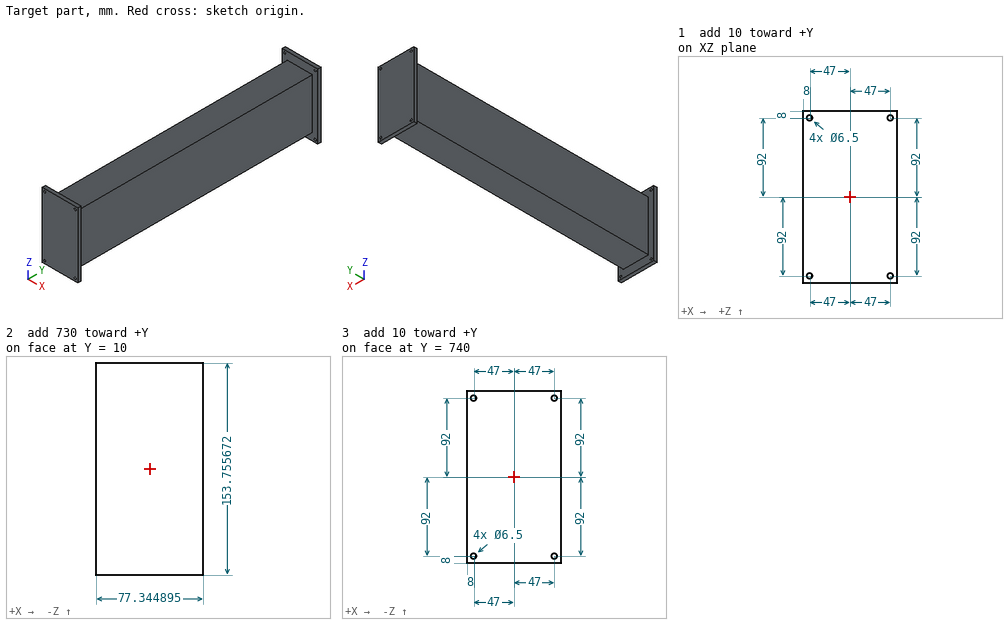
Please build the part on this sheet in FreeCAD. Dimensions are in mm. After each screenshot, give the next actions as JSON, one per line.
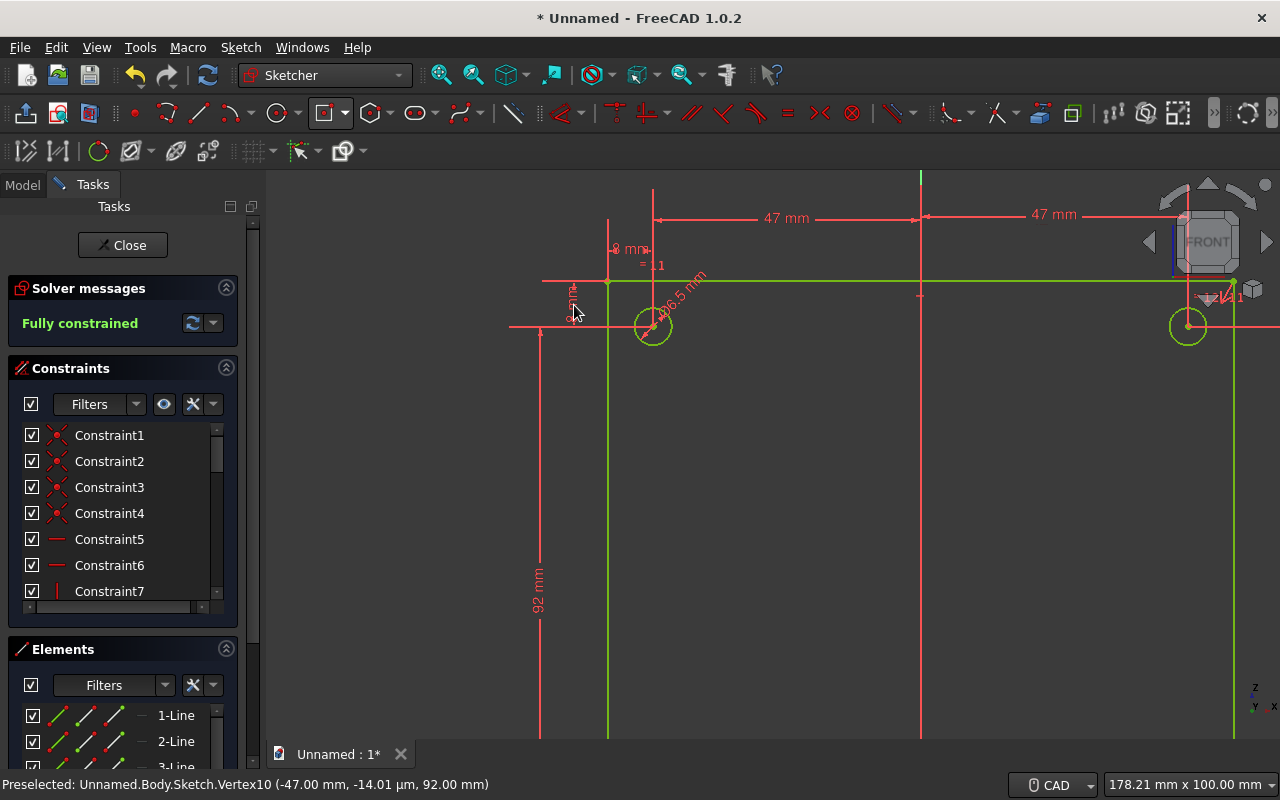
{"action": "left_click", "coordinate": [123, 245]}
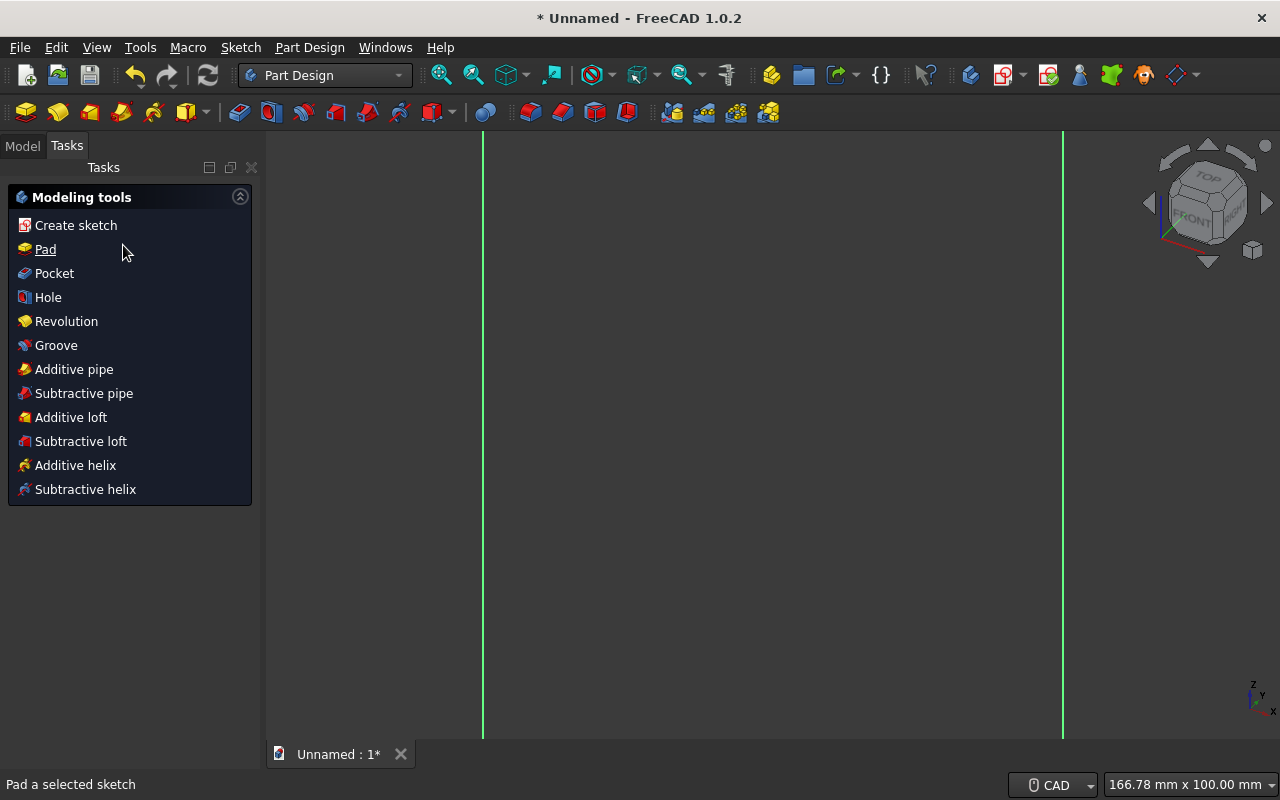
{"action": "left_click", "coordinate": [26, 112]}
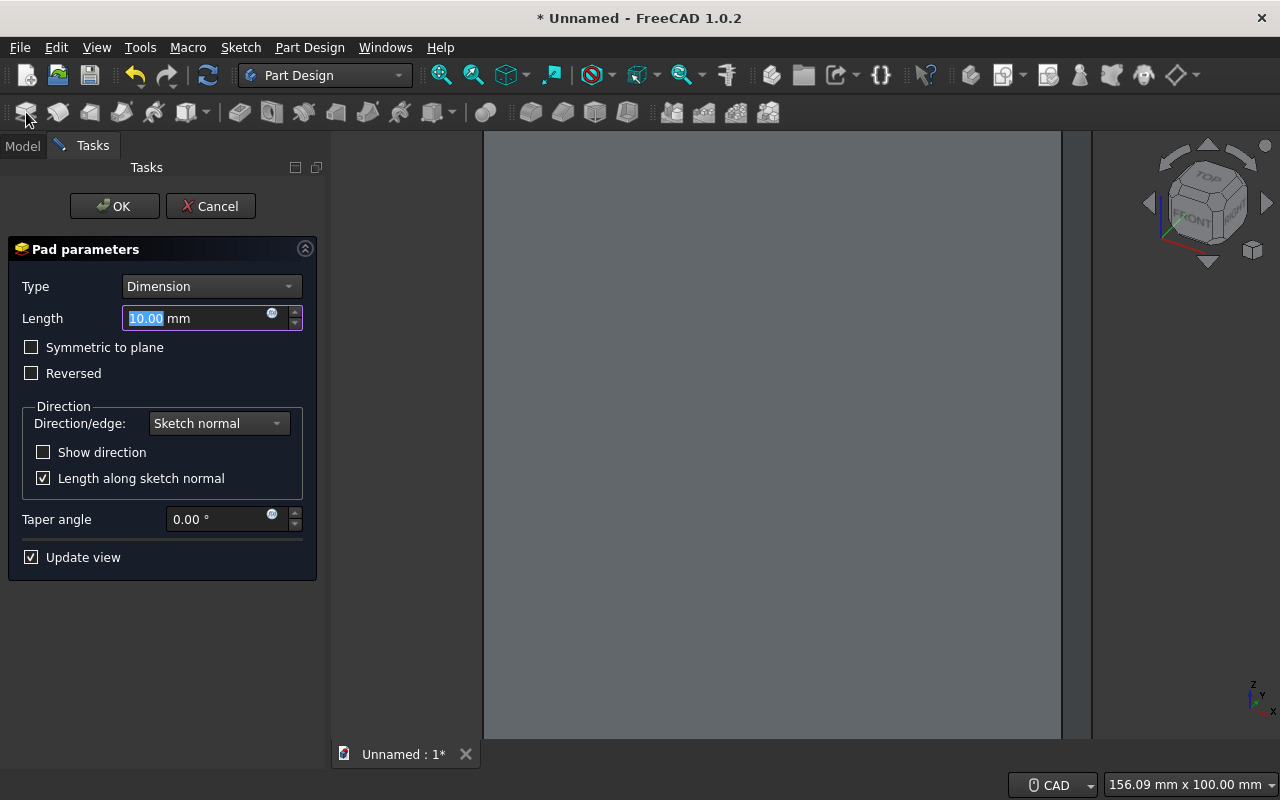
{"action": "type", "text": "10"}
{"action": "key", "text": "Tab"}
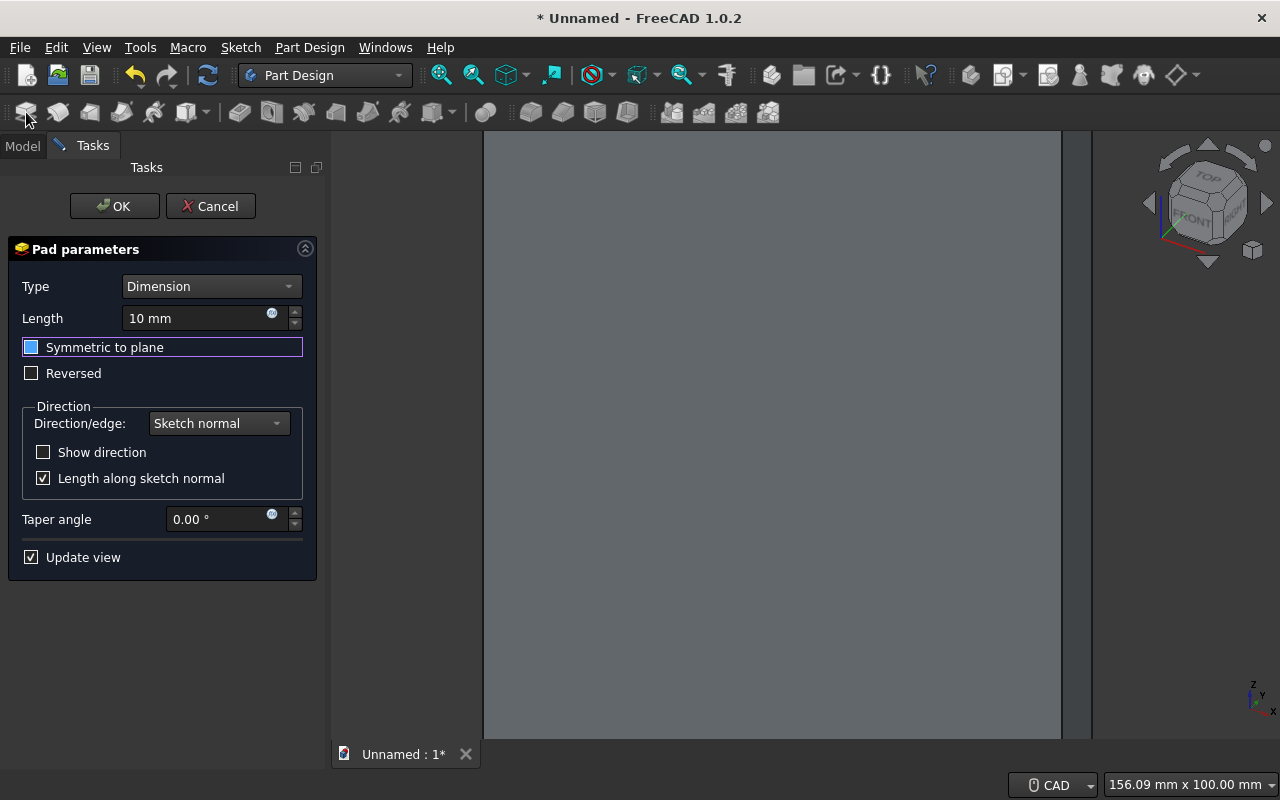
{"action": "left_click", "coordinate": [30, 373]}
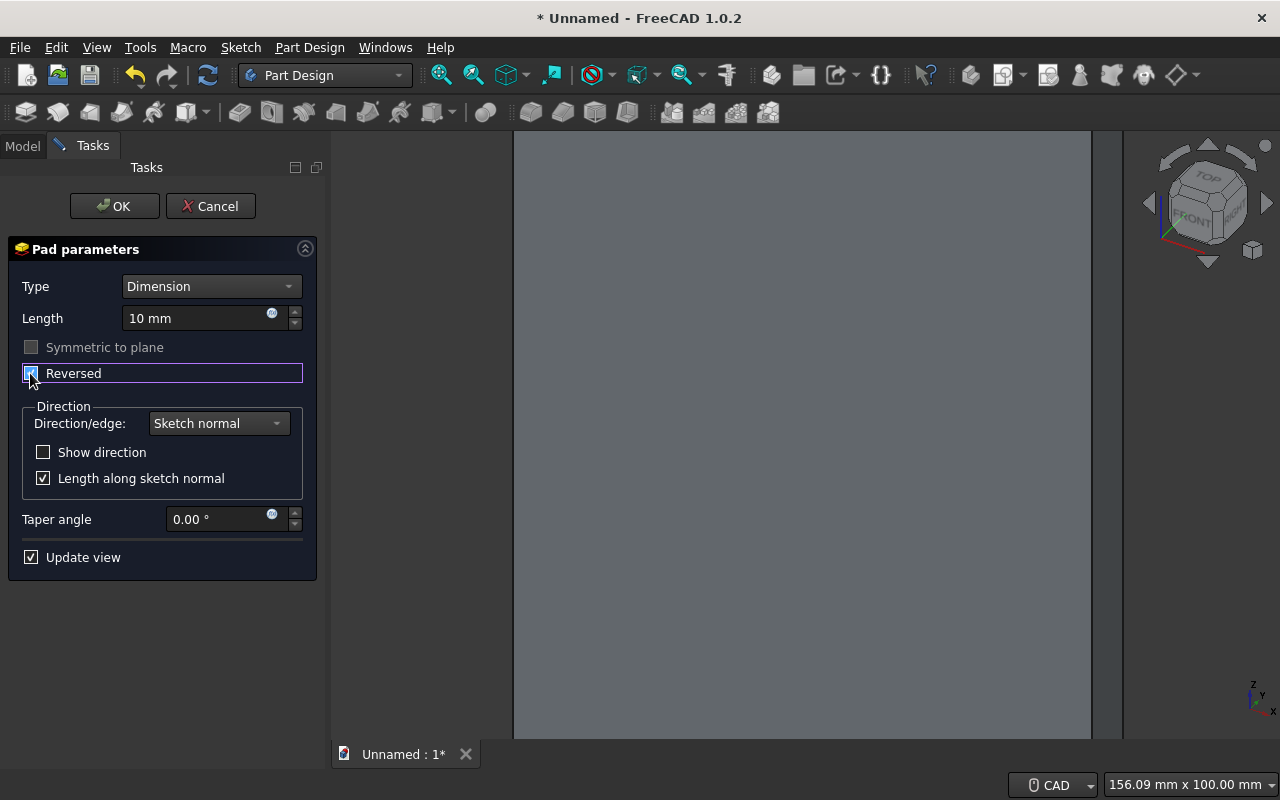
{"action": "left_click", "coordinate": [115, 206]}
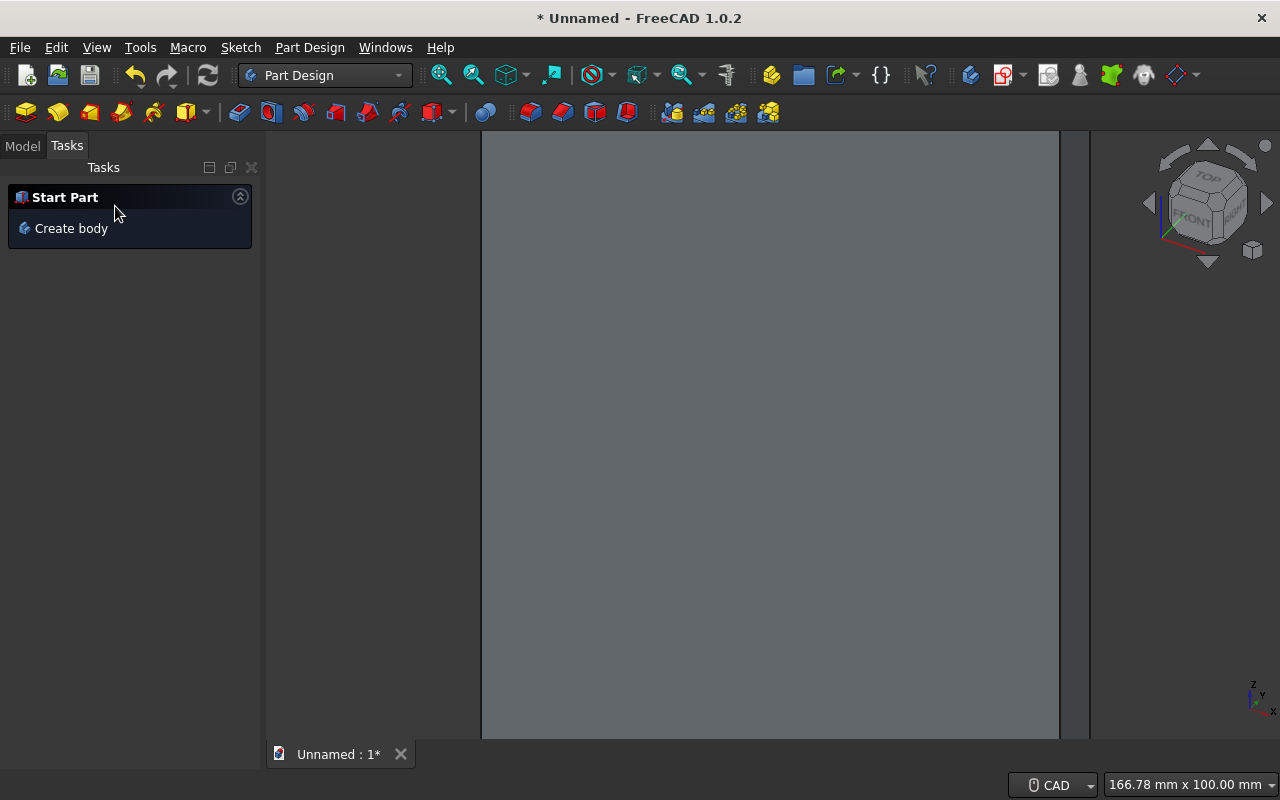
{"action": "left_click", "coordinate": [442, 76]}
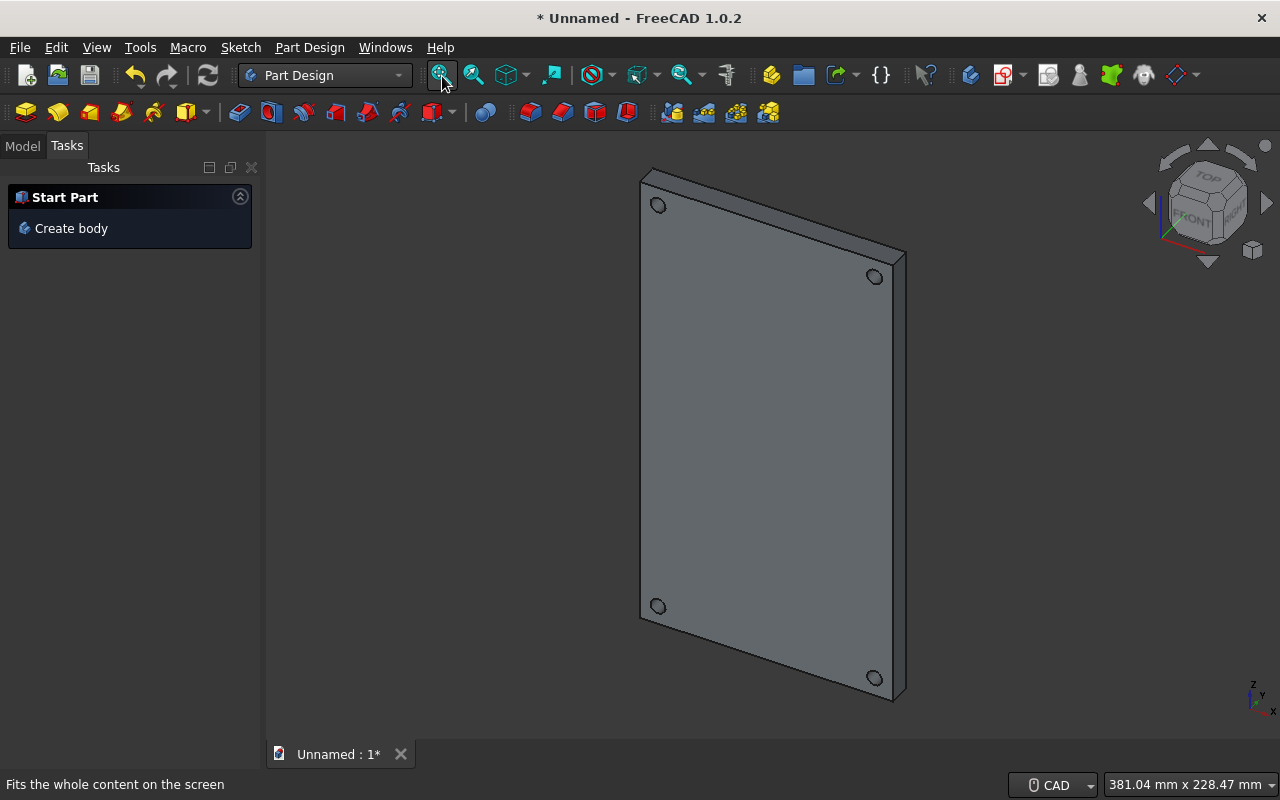
{"action": "key", "text": "4"}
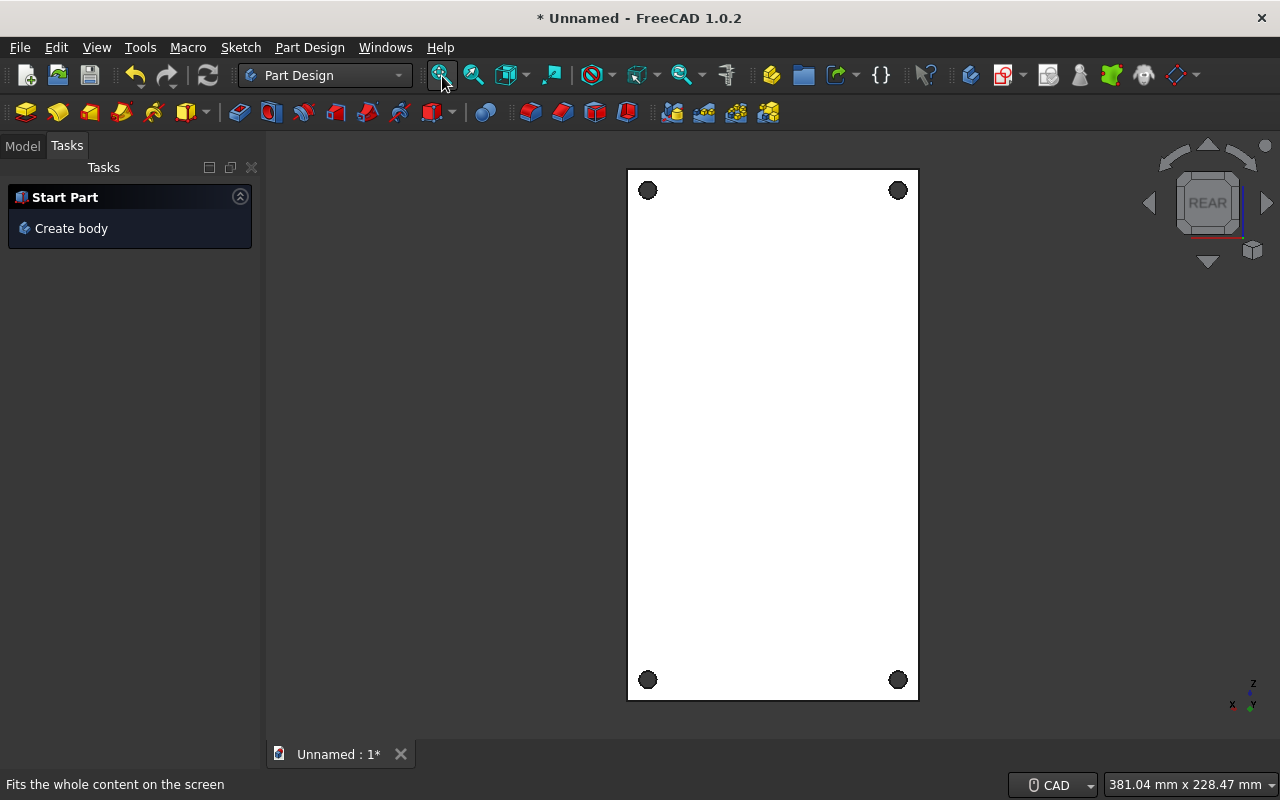
{"action": "left_click", "coordinate": [773, 358]}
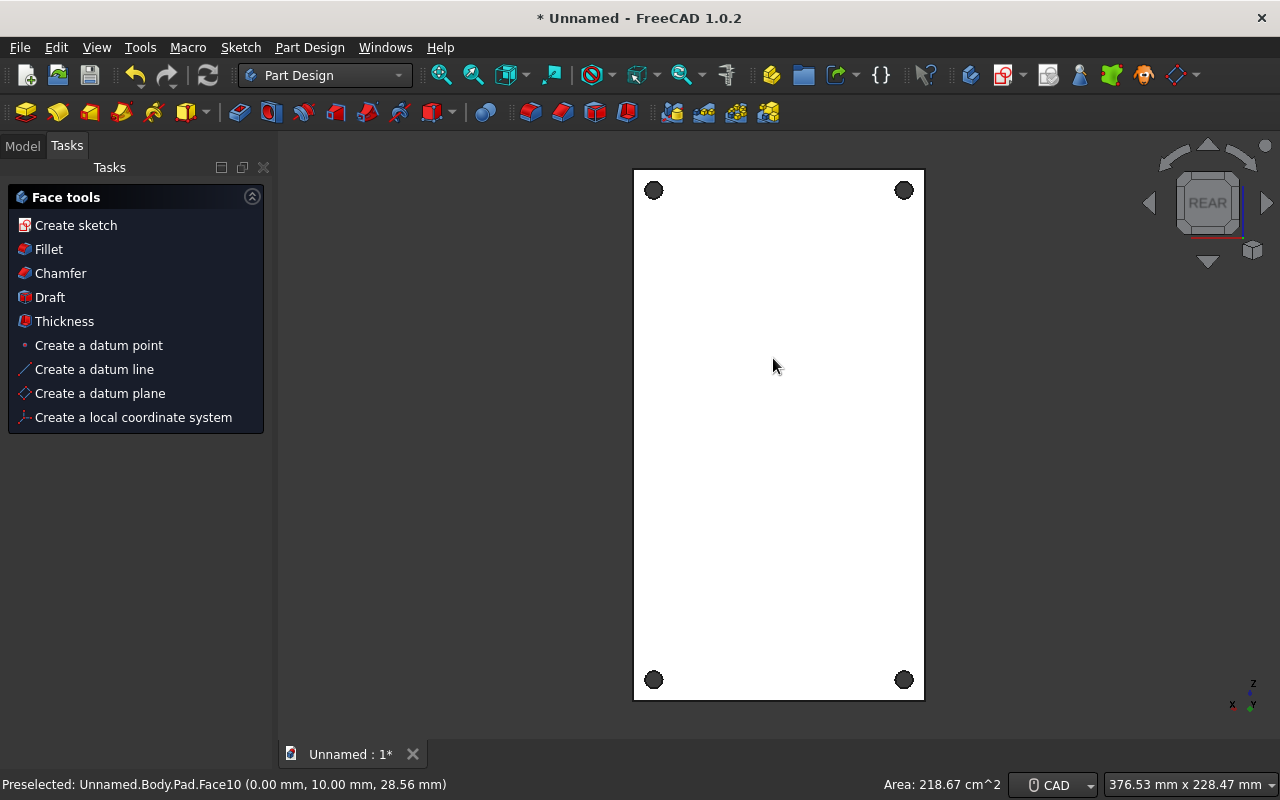
{"action": "left_click", "coordinate": [1004, 76]}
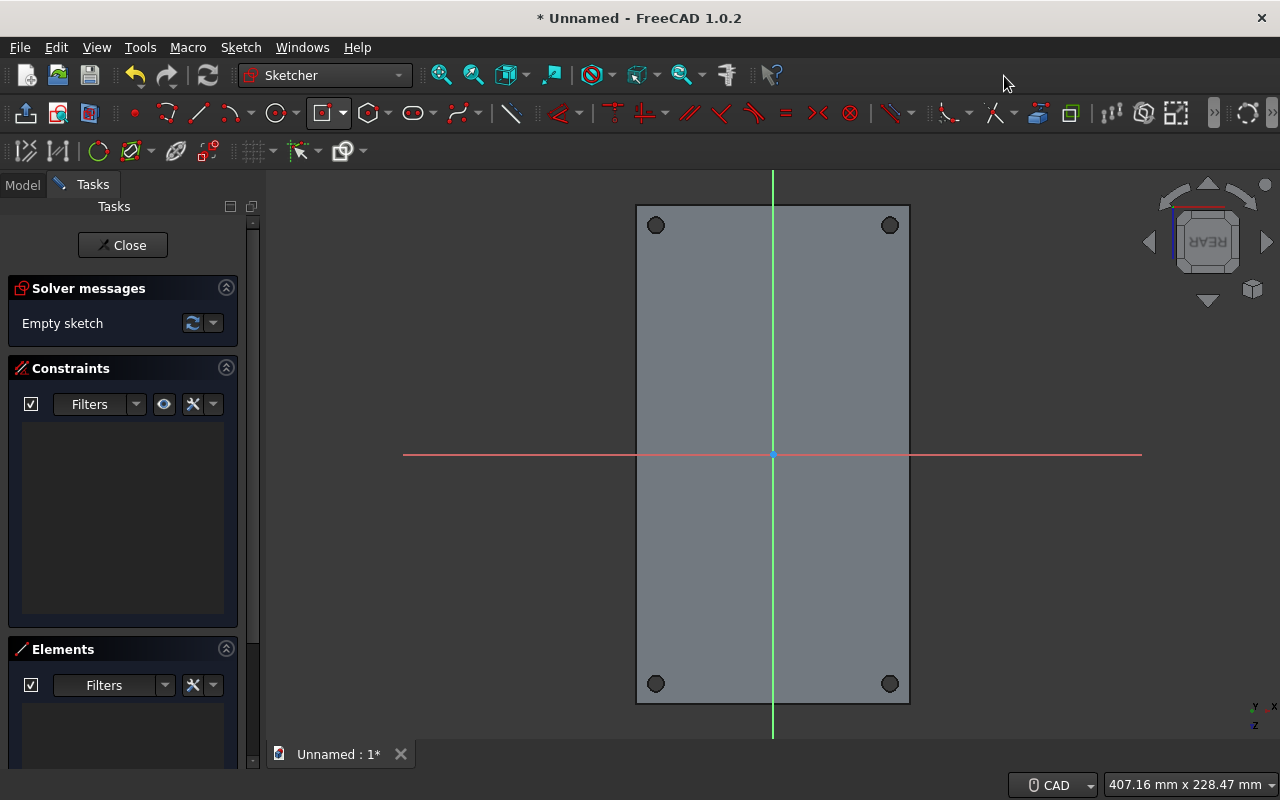
{"action": "left_click", "coordinate": [322, 114]}